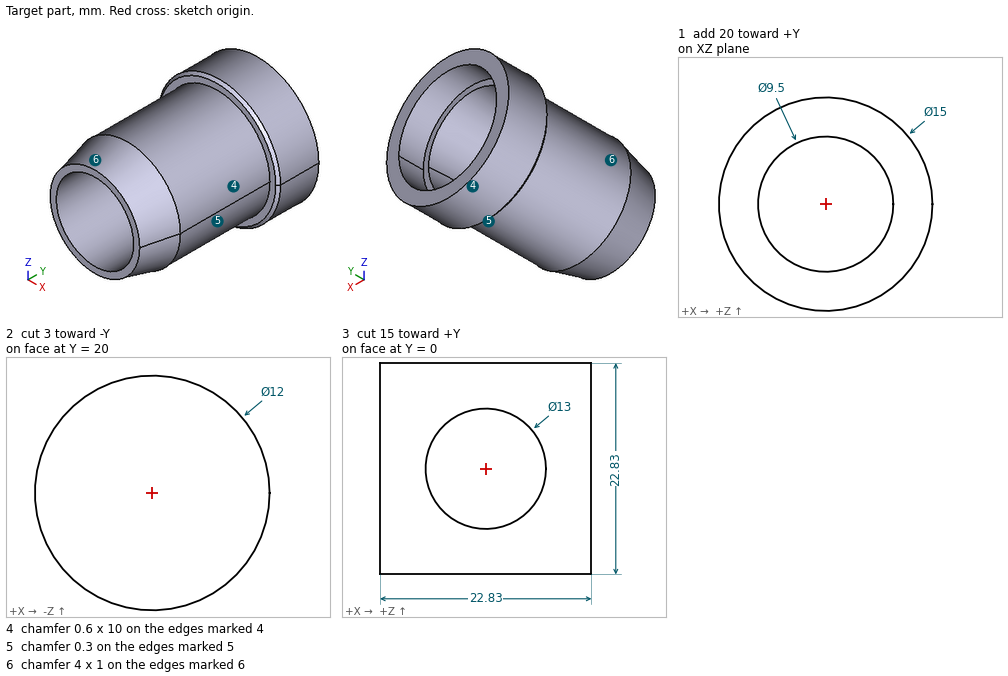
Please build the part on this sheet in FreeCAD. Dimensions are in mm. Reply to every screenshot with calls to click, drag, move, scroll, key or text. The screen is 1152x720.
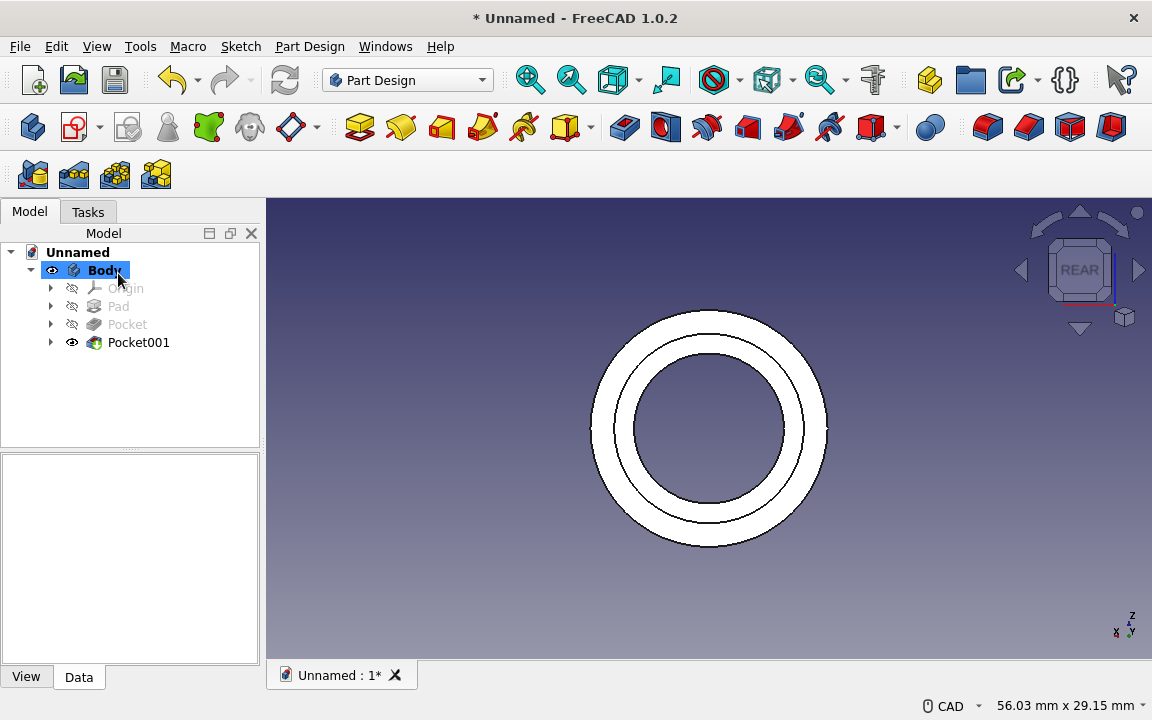
click(770, 383)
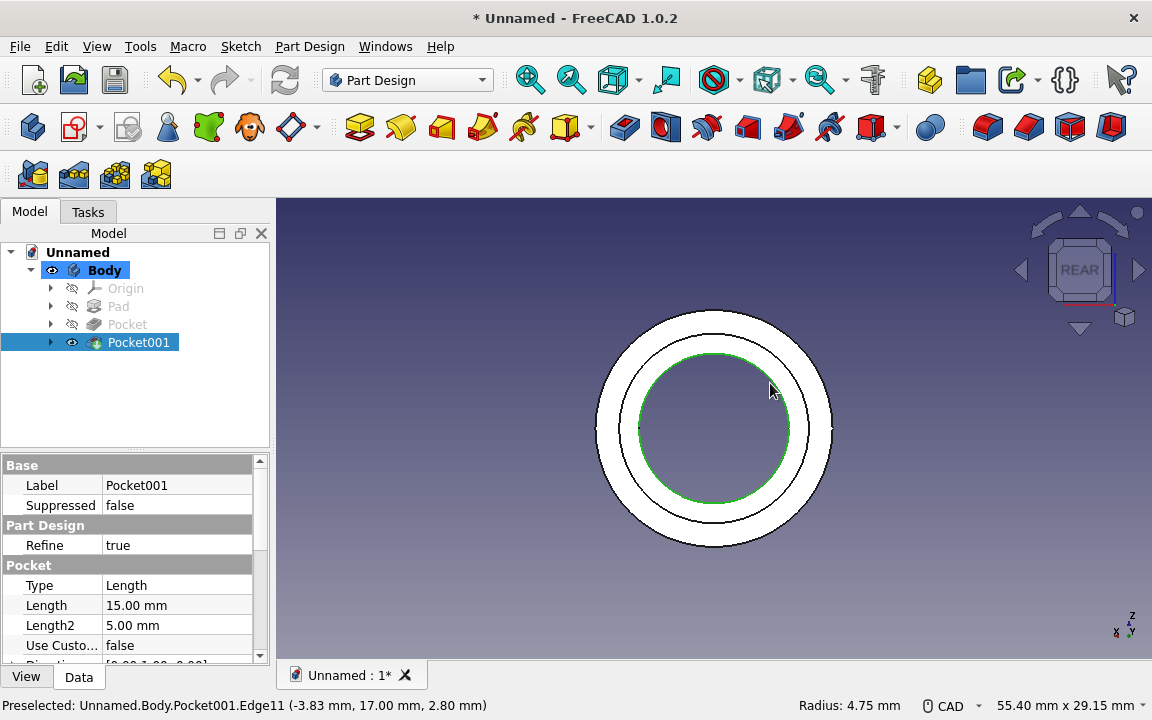
click(1029, 128)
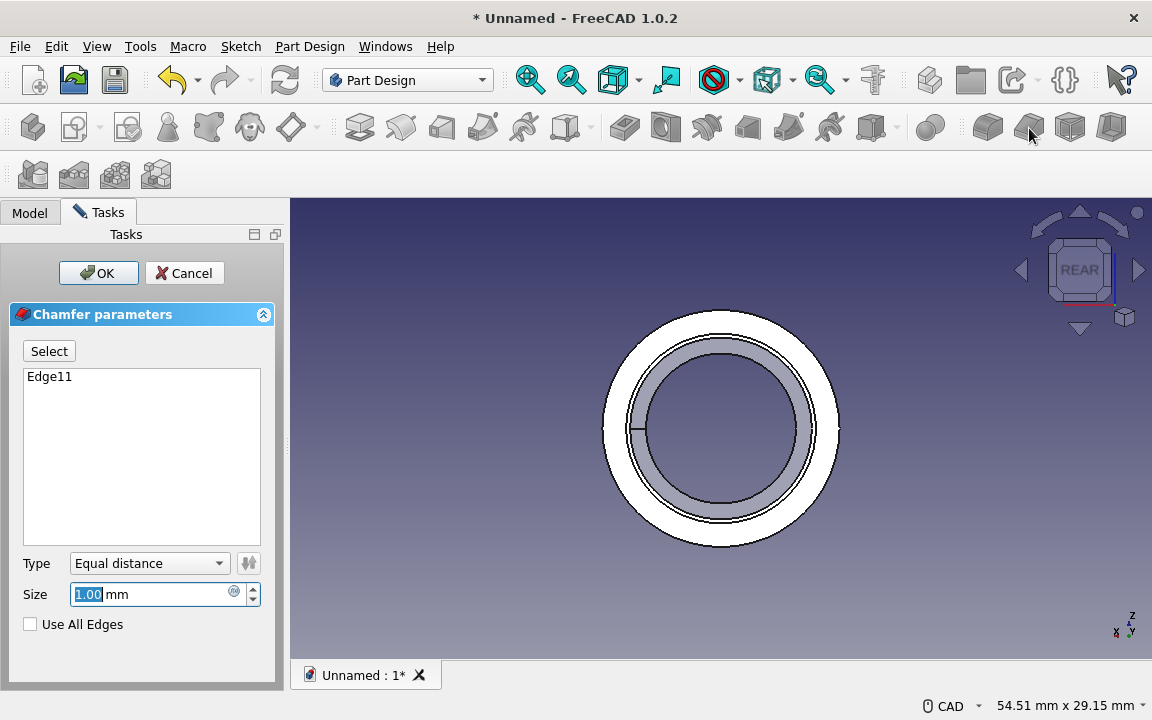
text(0.6)
key(Tab)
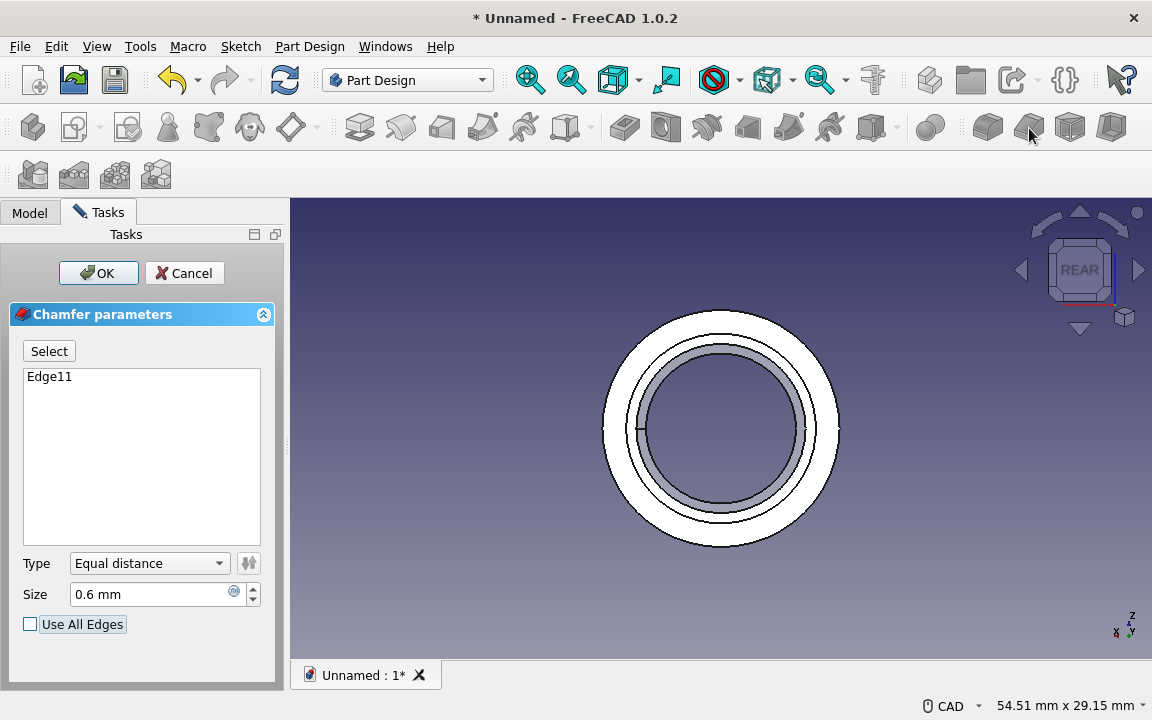
click(150, 564)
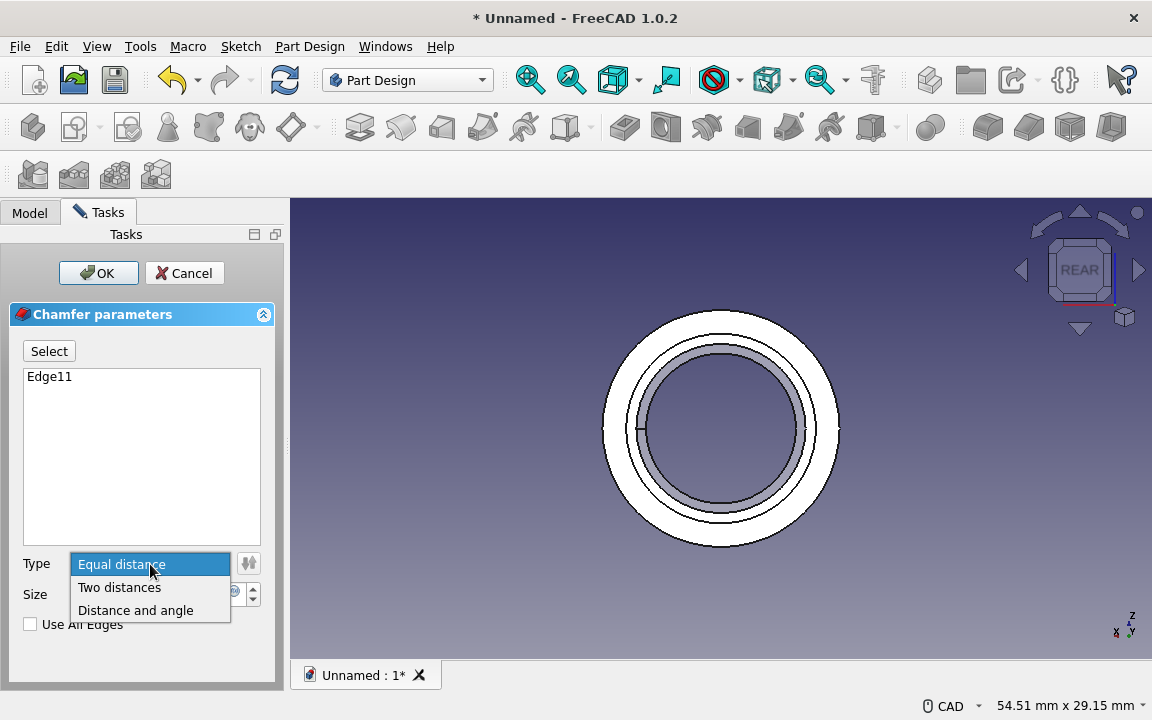
click(148, 588)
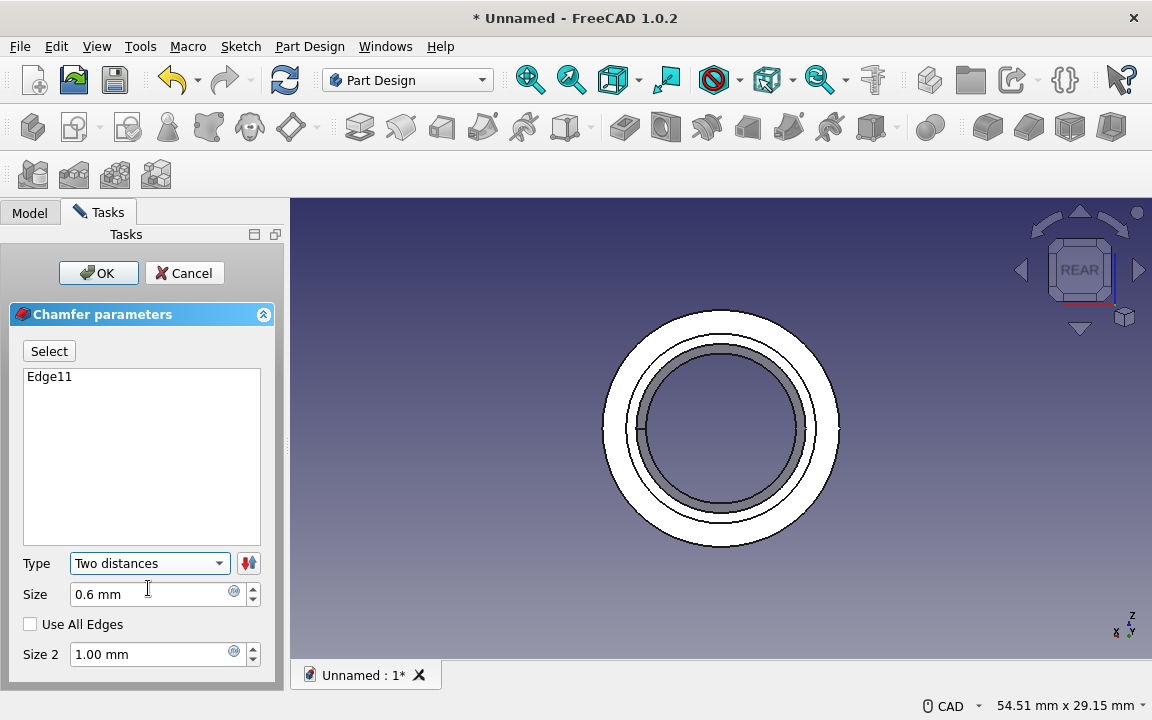
triple_click(158, 654)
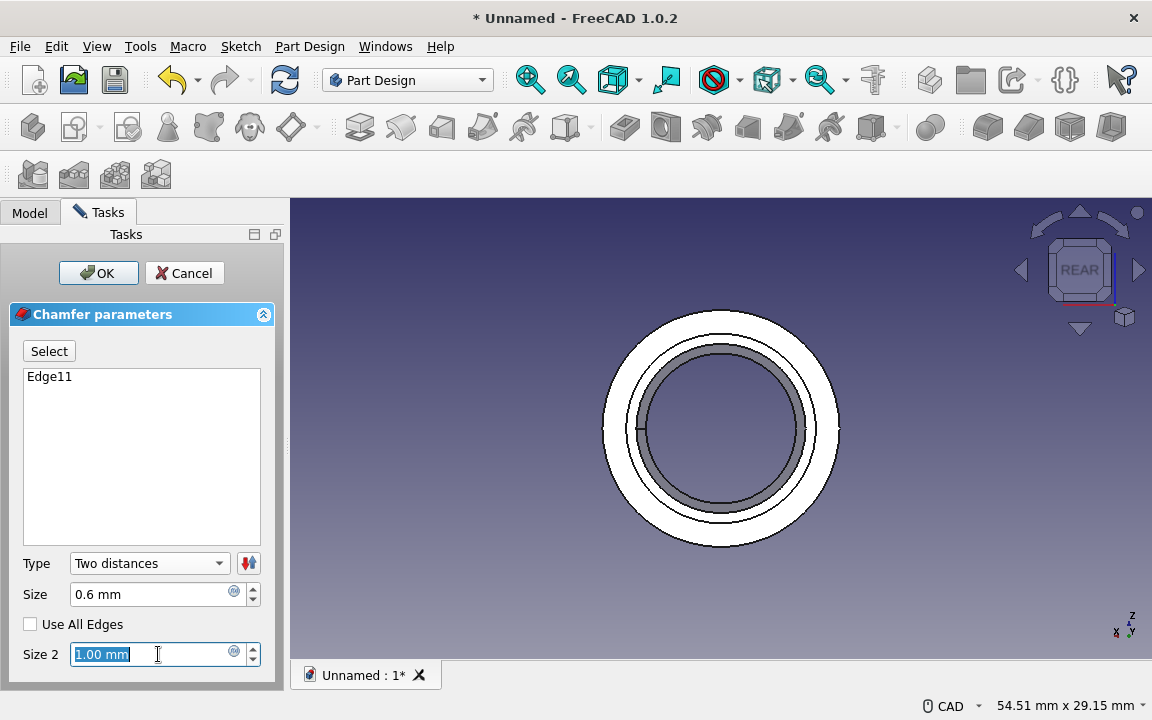
text(10)
key(Tab)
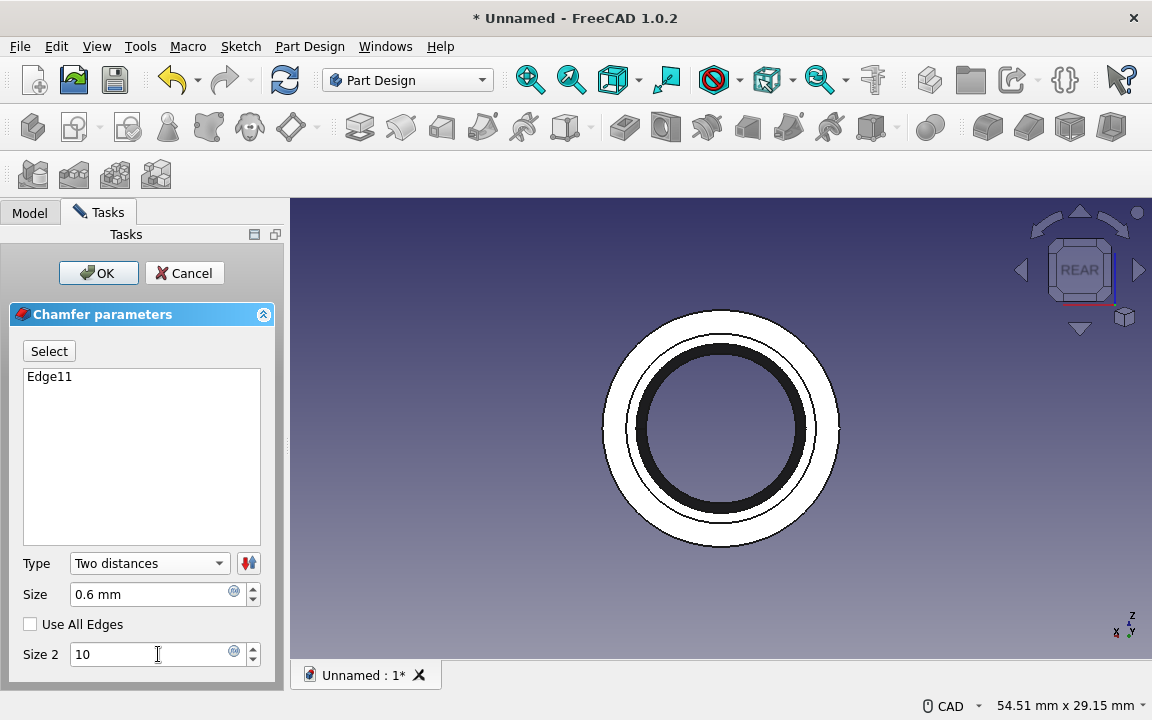
click(99, 273)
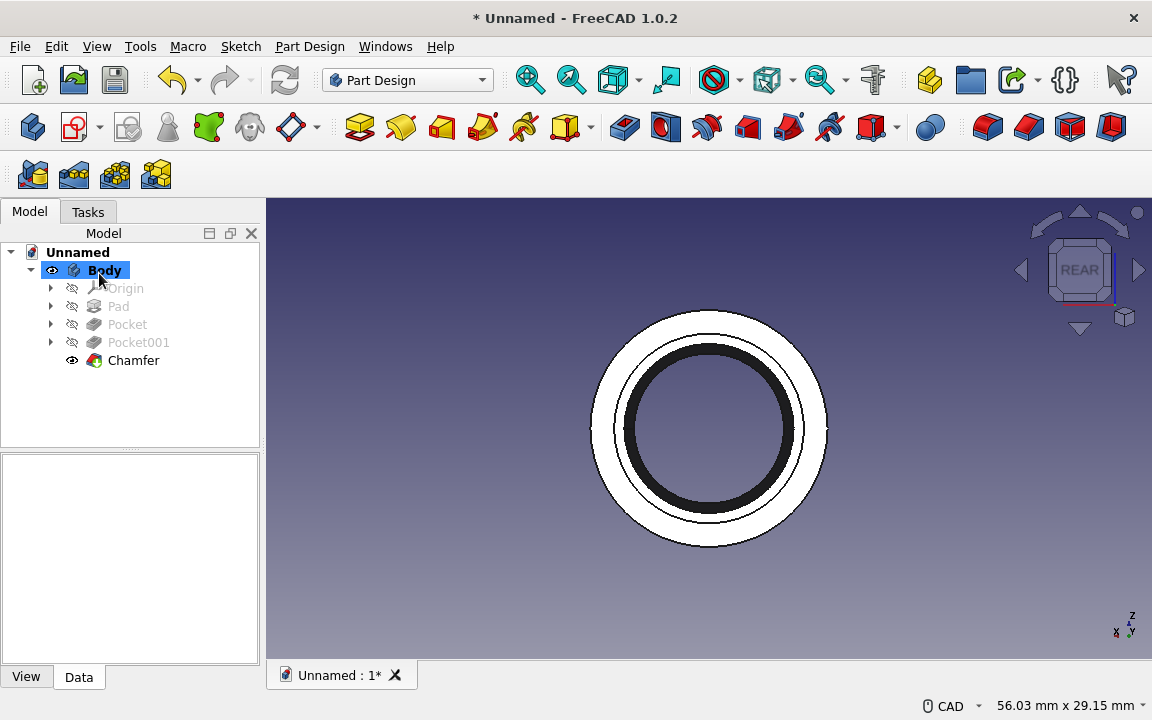
key(0)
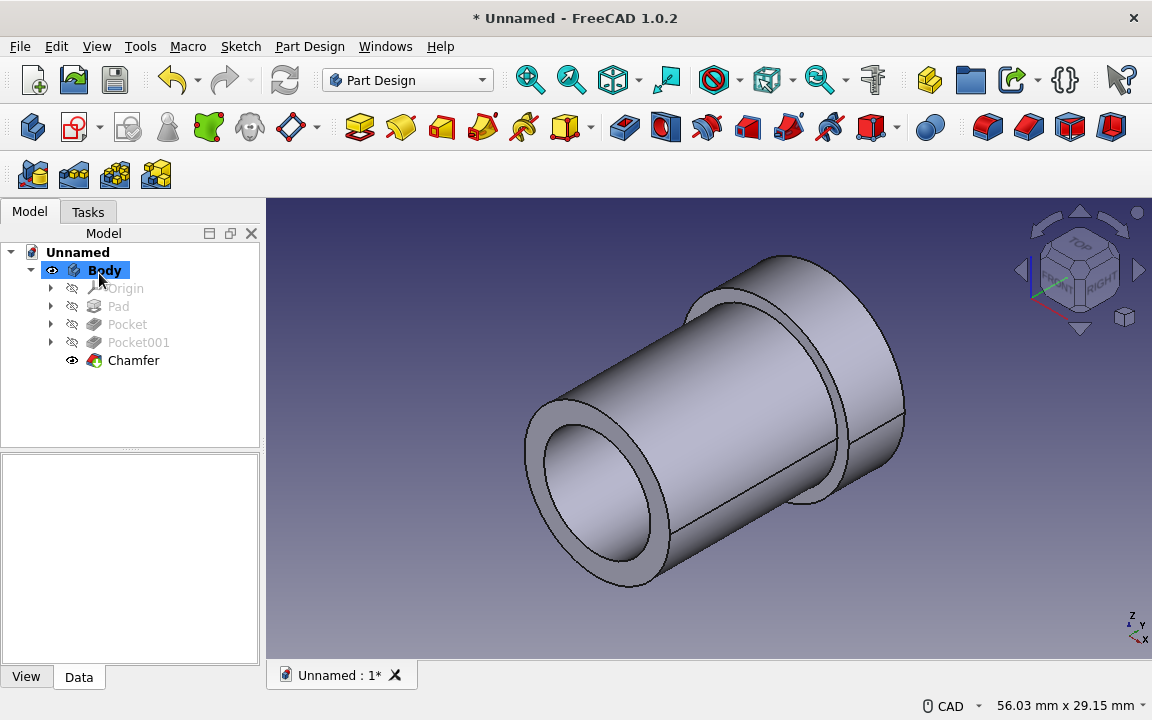
click(697, 299)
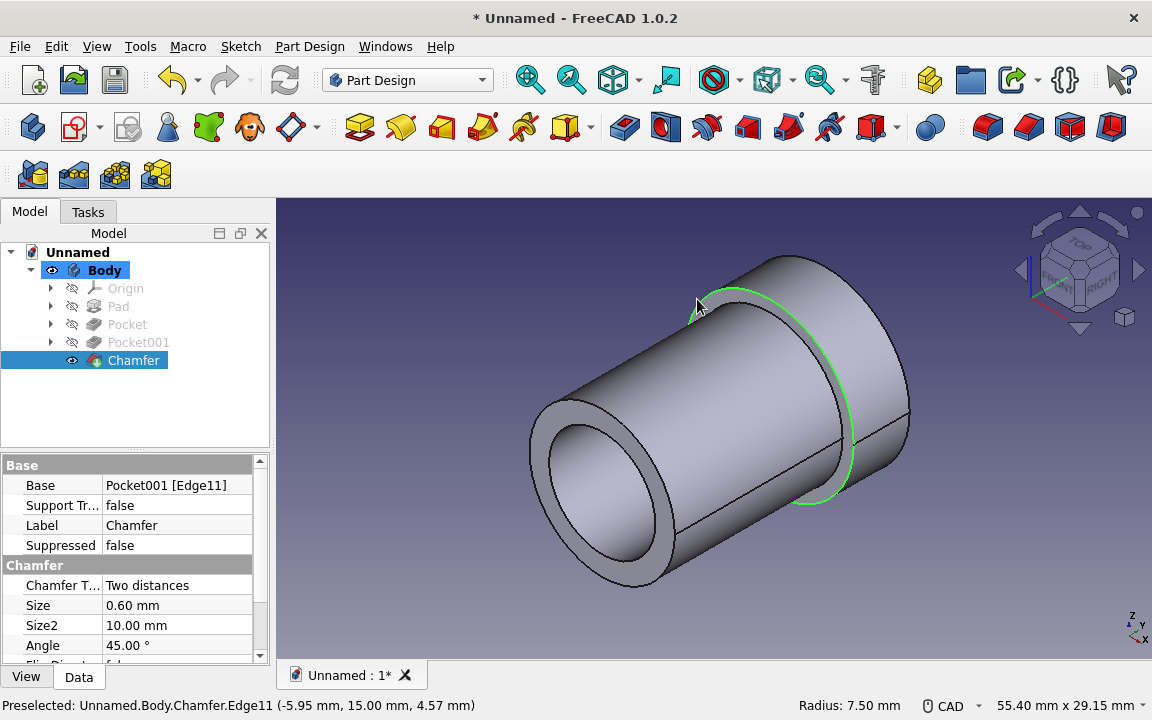
click(1029, 128)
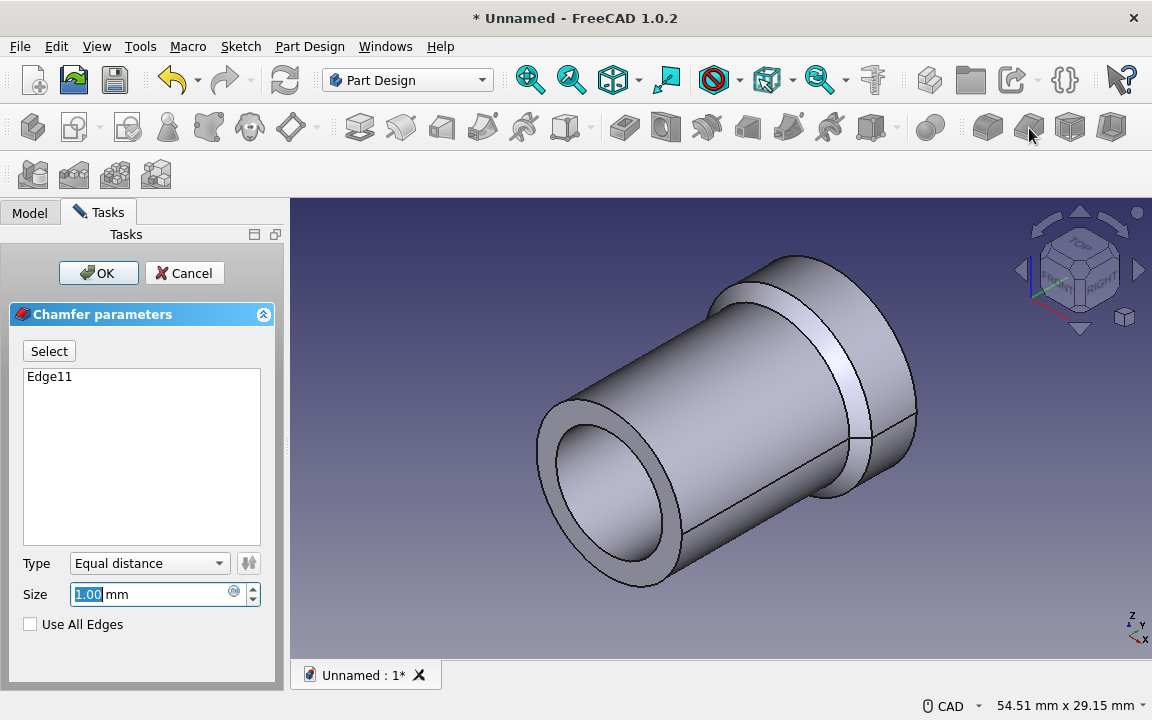
text(0.3)
key(Tab)